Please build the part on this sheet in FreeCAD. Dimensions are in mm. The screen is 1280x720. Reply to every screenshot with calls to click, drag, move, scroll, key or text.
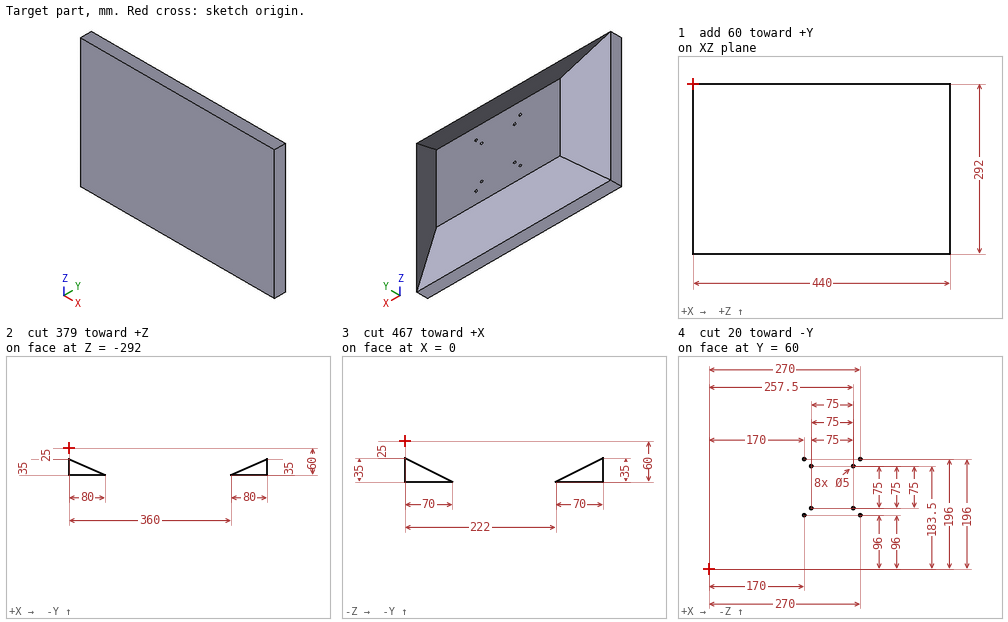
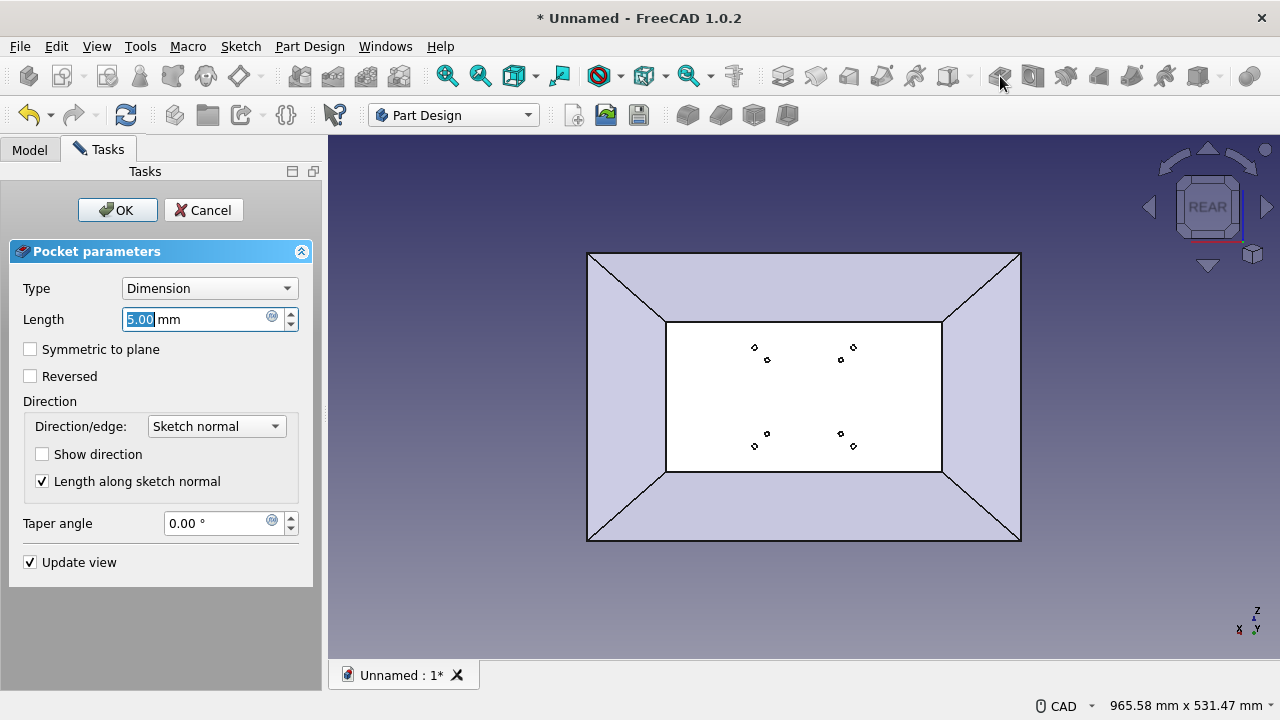
text(20)
key(Tab)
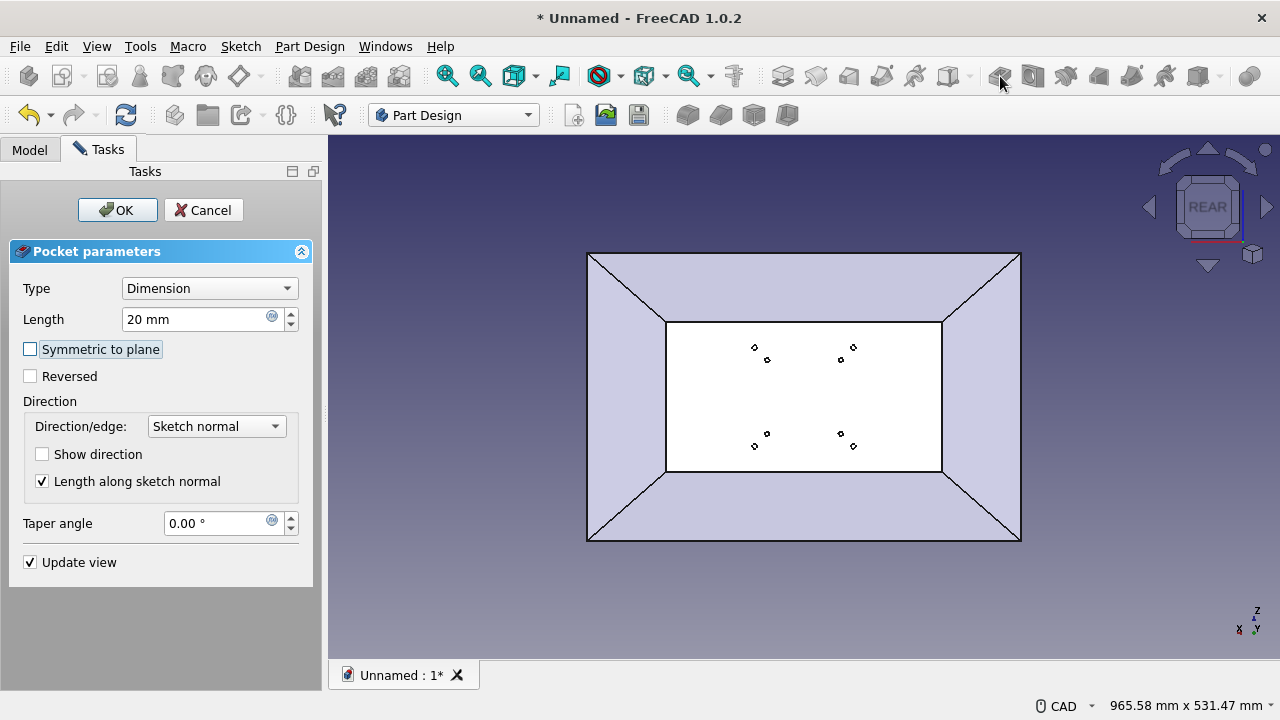
click(118, 210)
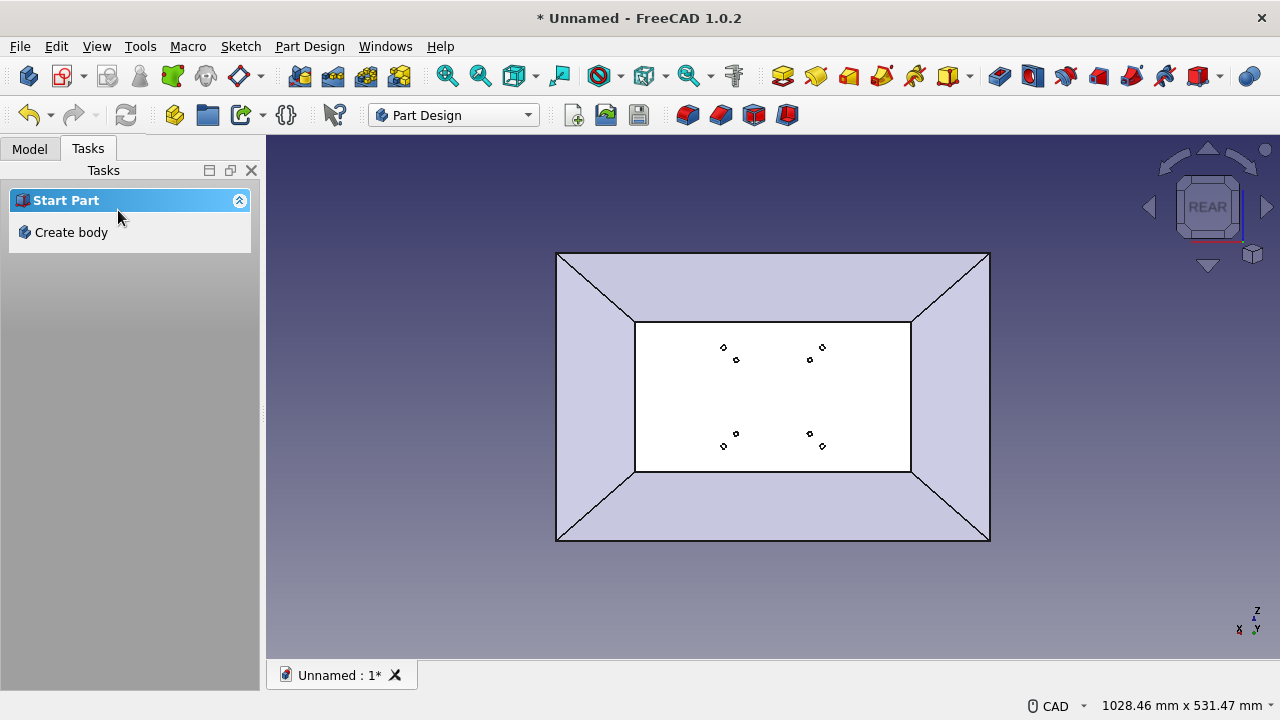
key(0)